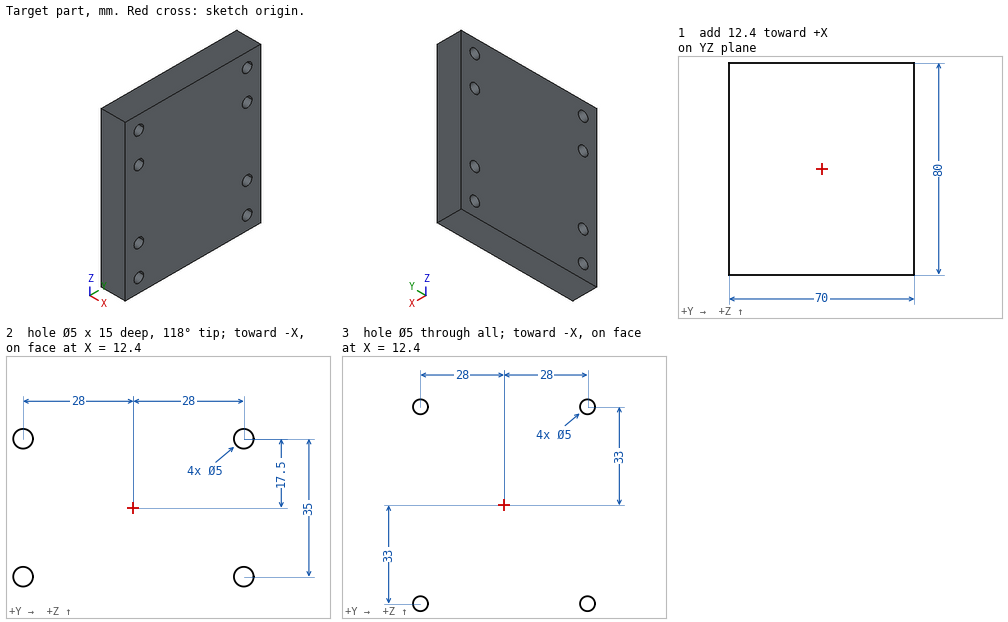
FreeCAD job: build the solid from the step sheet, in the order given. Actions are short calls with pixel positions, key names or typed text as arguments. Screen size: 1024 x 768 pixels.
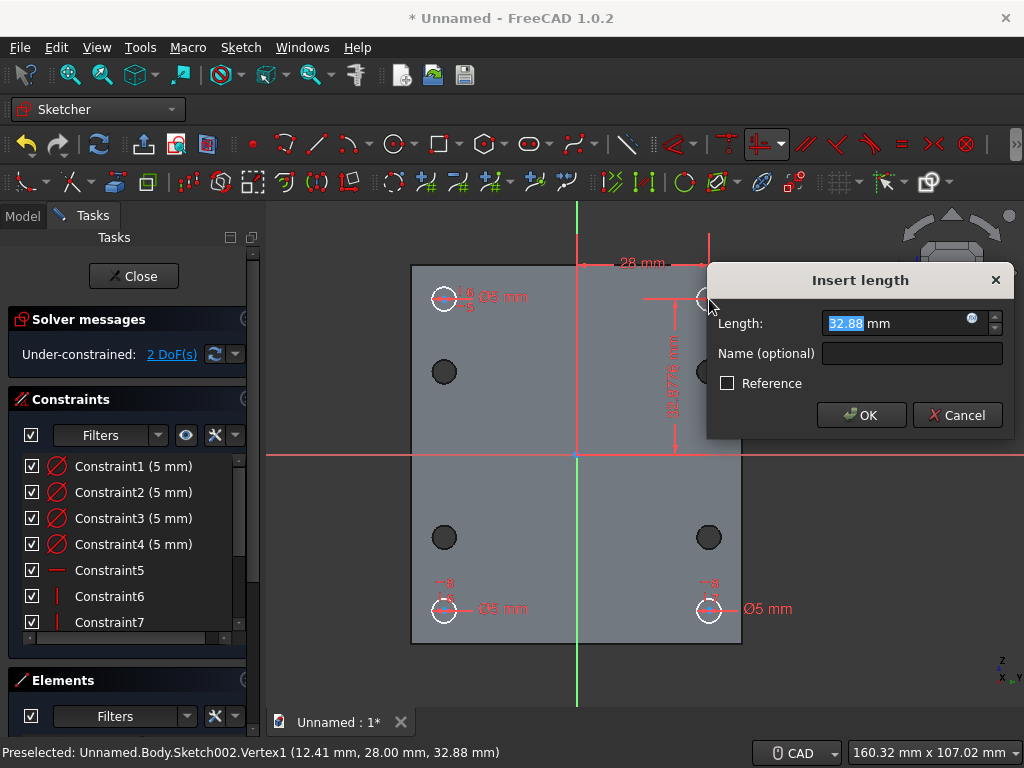
text(33)
key(Return)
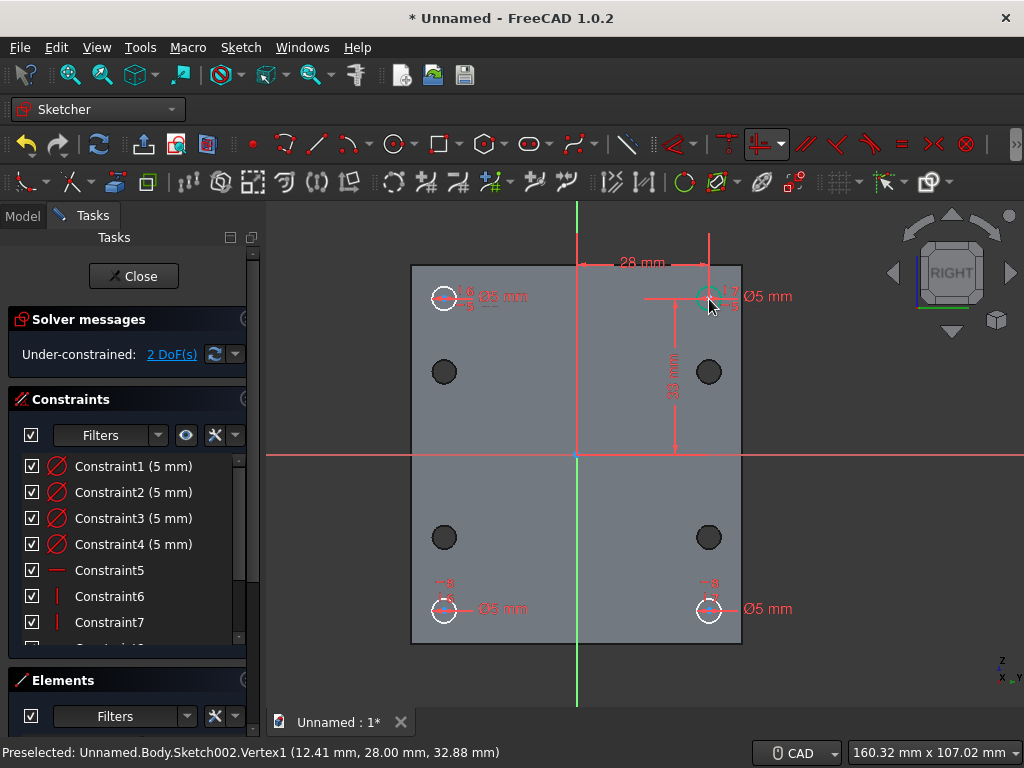
click(444, 299)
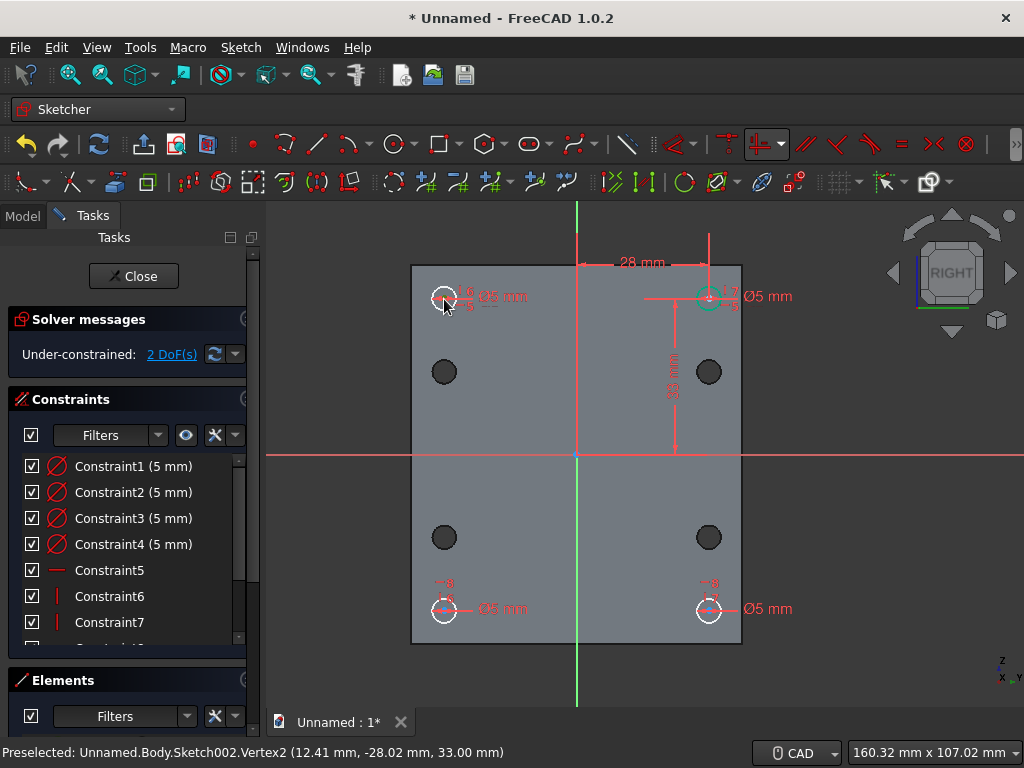
click(696, 144)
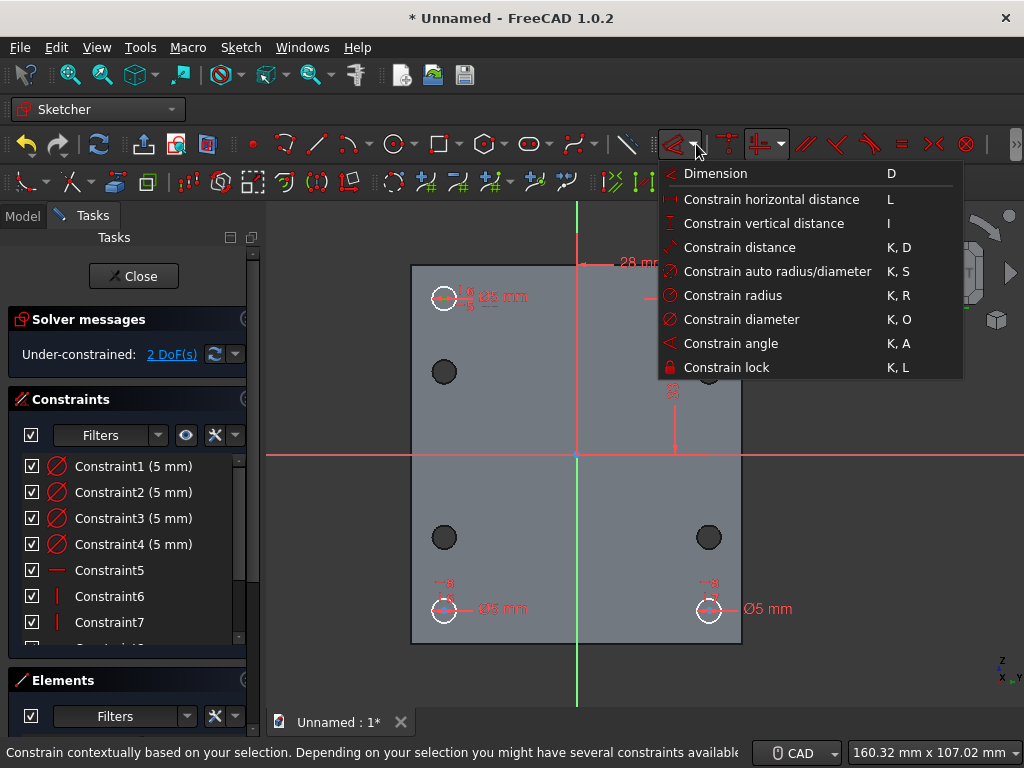
click(811, 199)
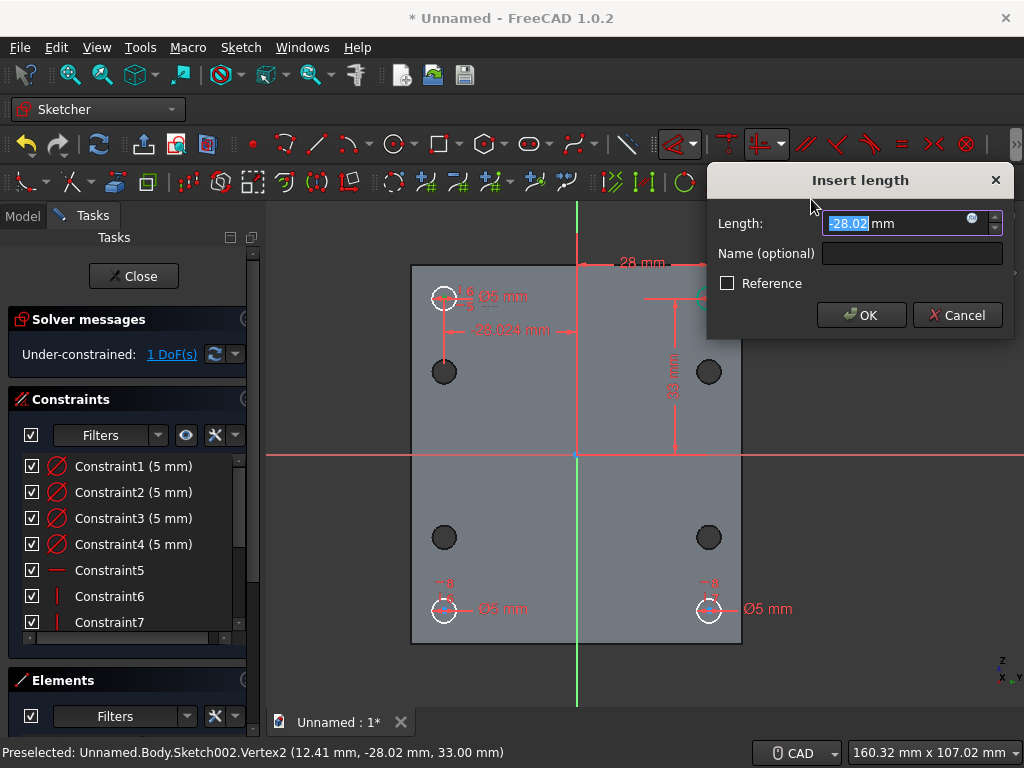
text(-28)
key(Return)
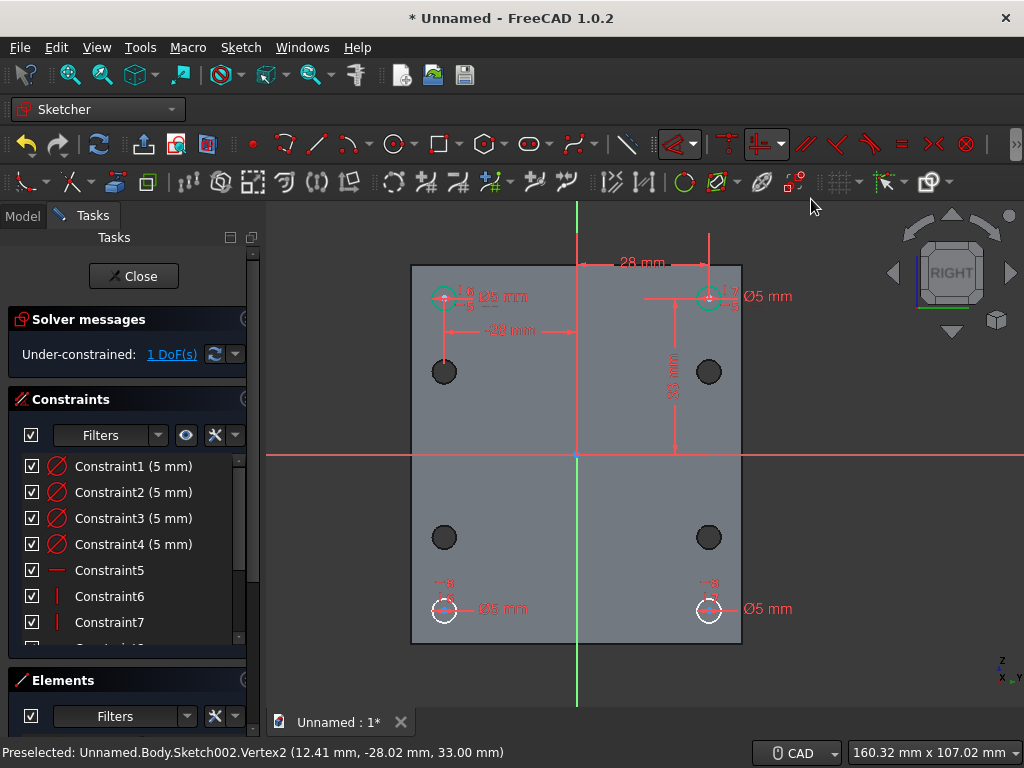
click(444, 611)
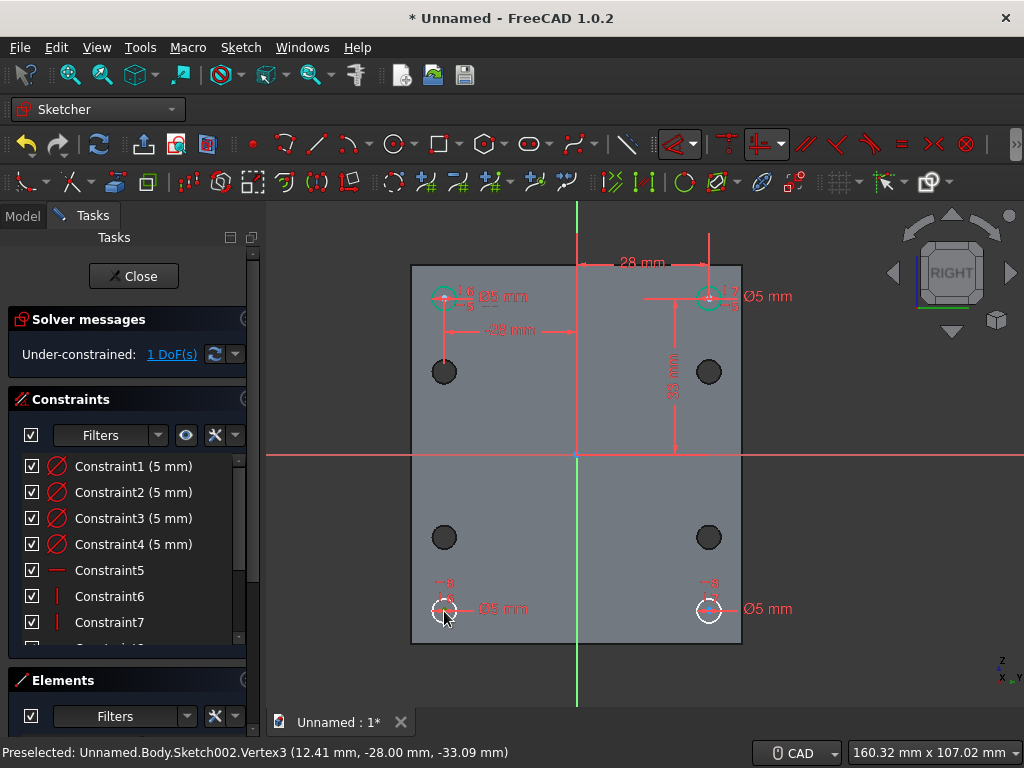
key(i)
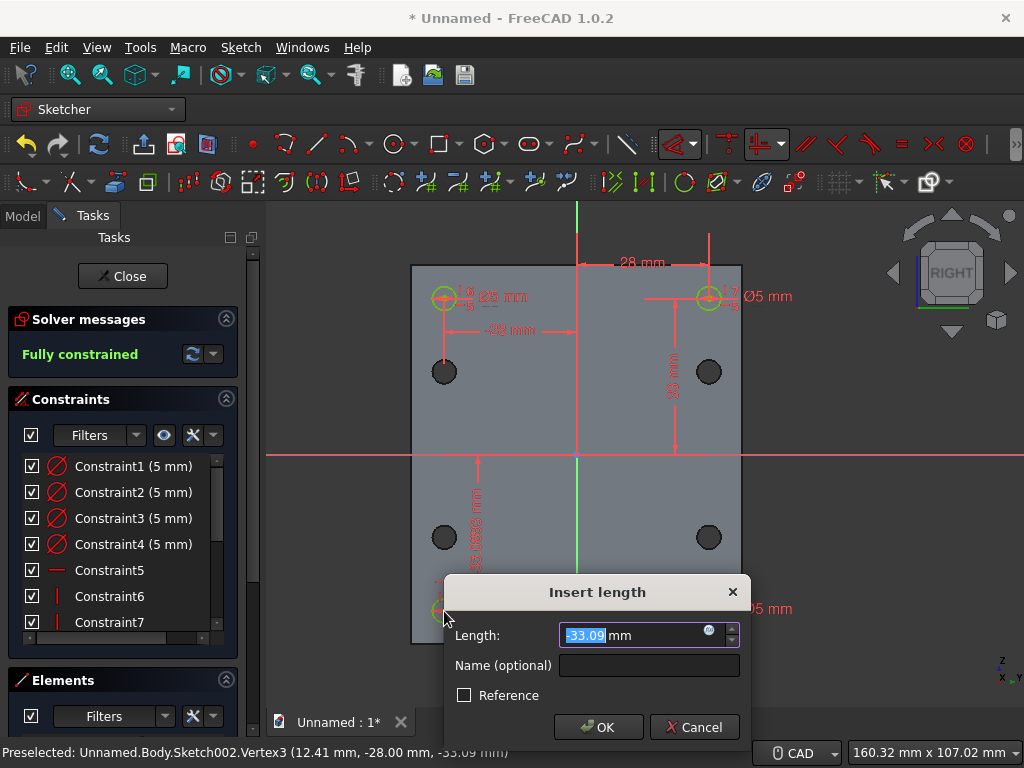
text(-33)
key(Return)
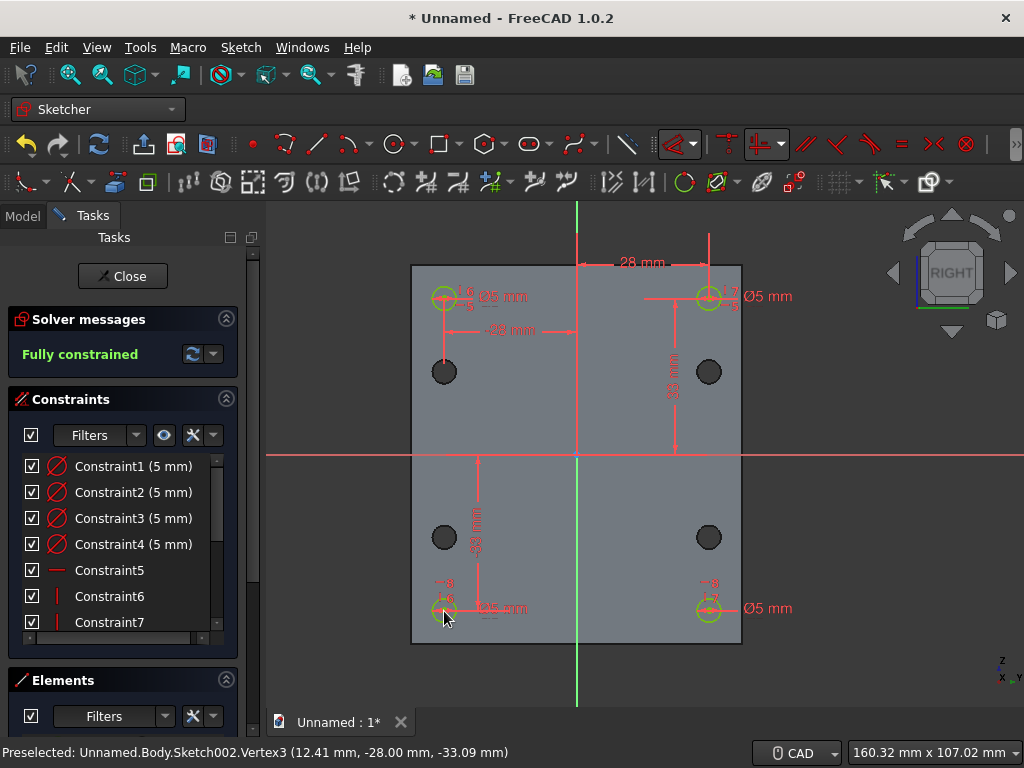
click(123, 276)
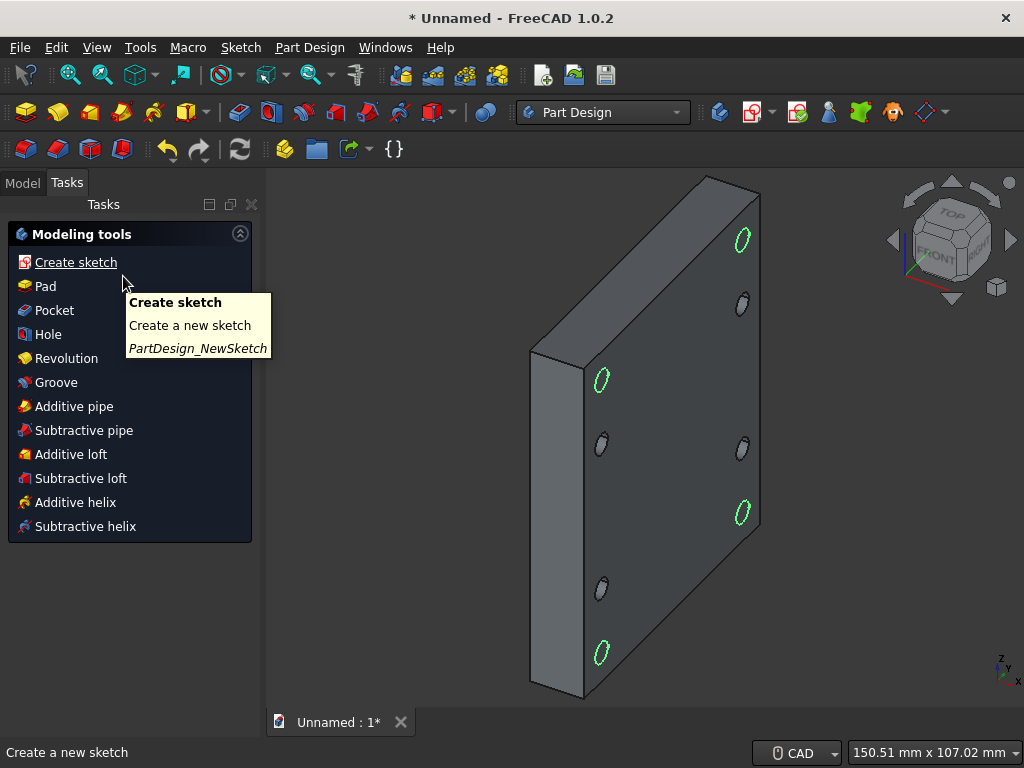
click(272, 112)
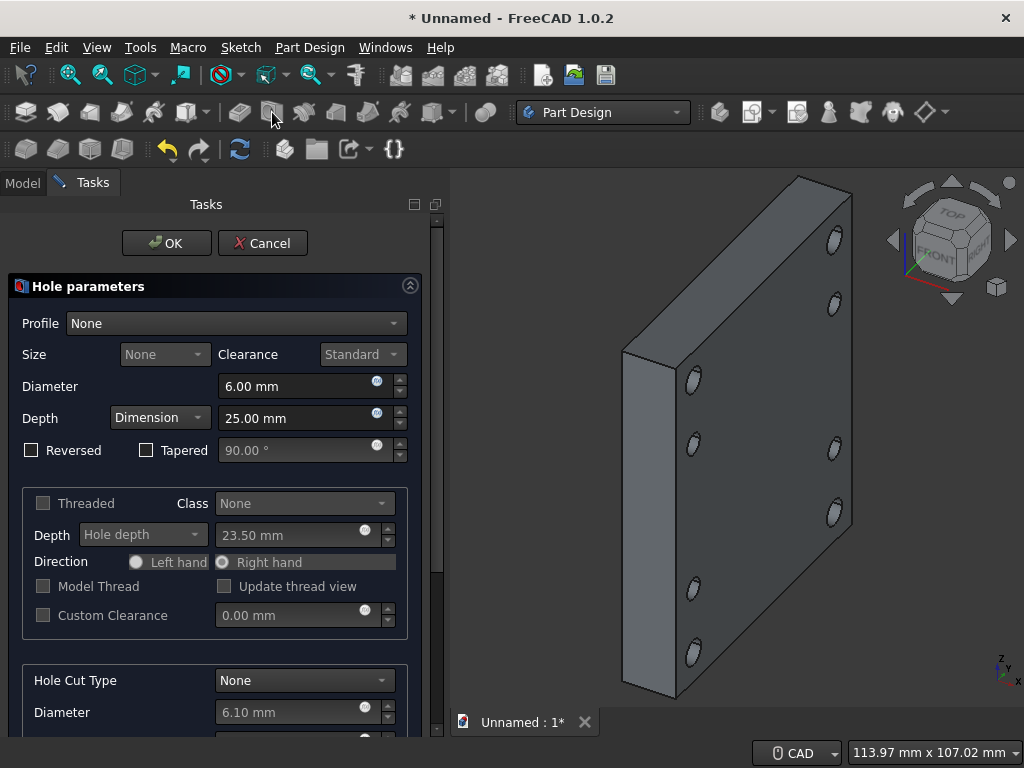
triple_click(305, 386)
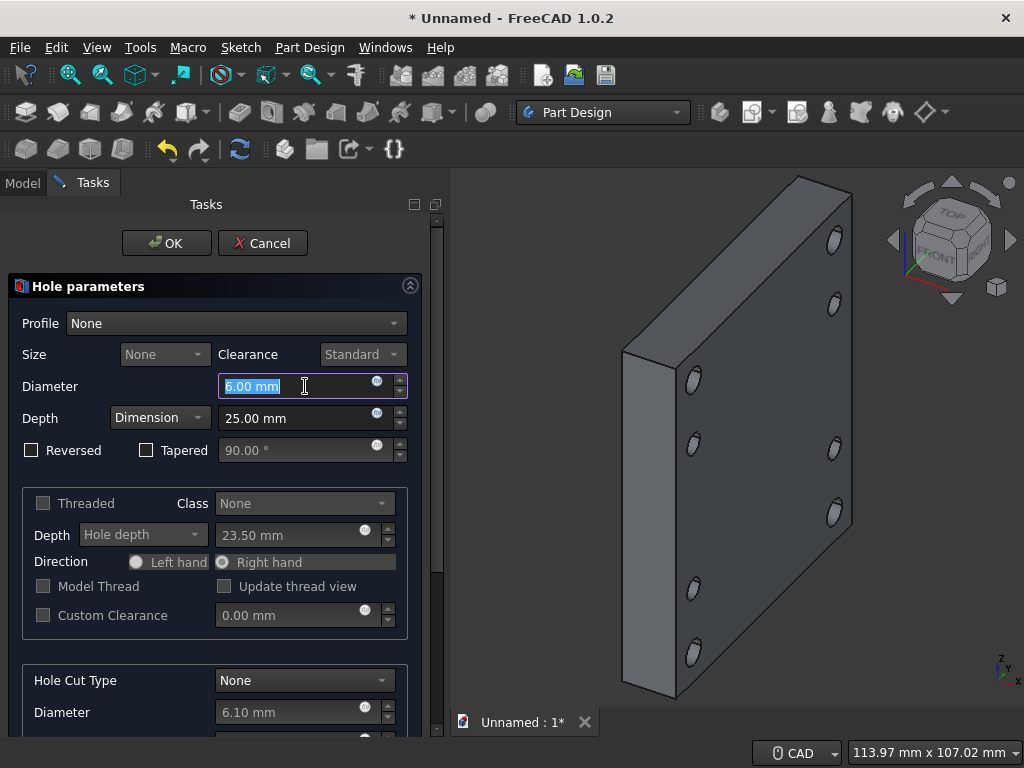
text(5)
key(Tab)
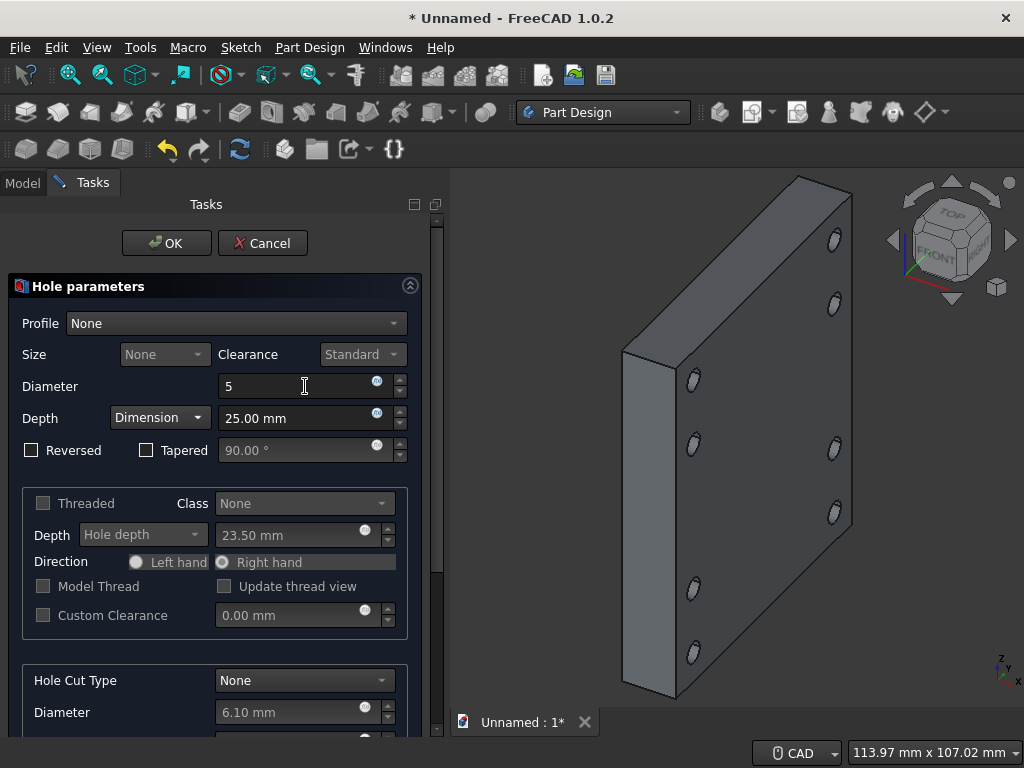
click(161, 418)